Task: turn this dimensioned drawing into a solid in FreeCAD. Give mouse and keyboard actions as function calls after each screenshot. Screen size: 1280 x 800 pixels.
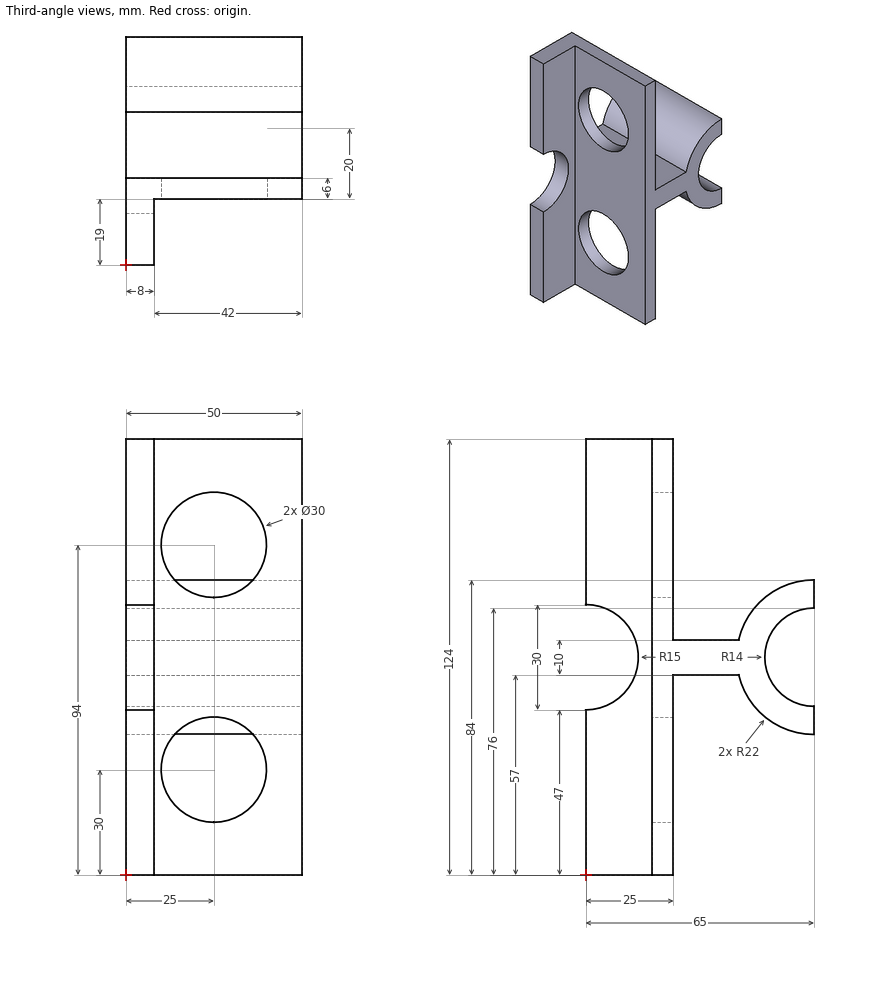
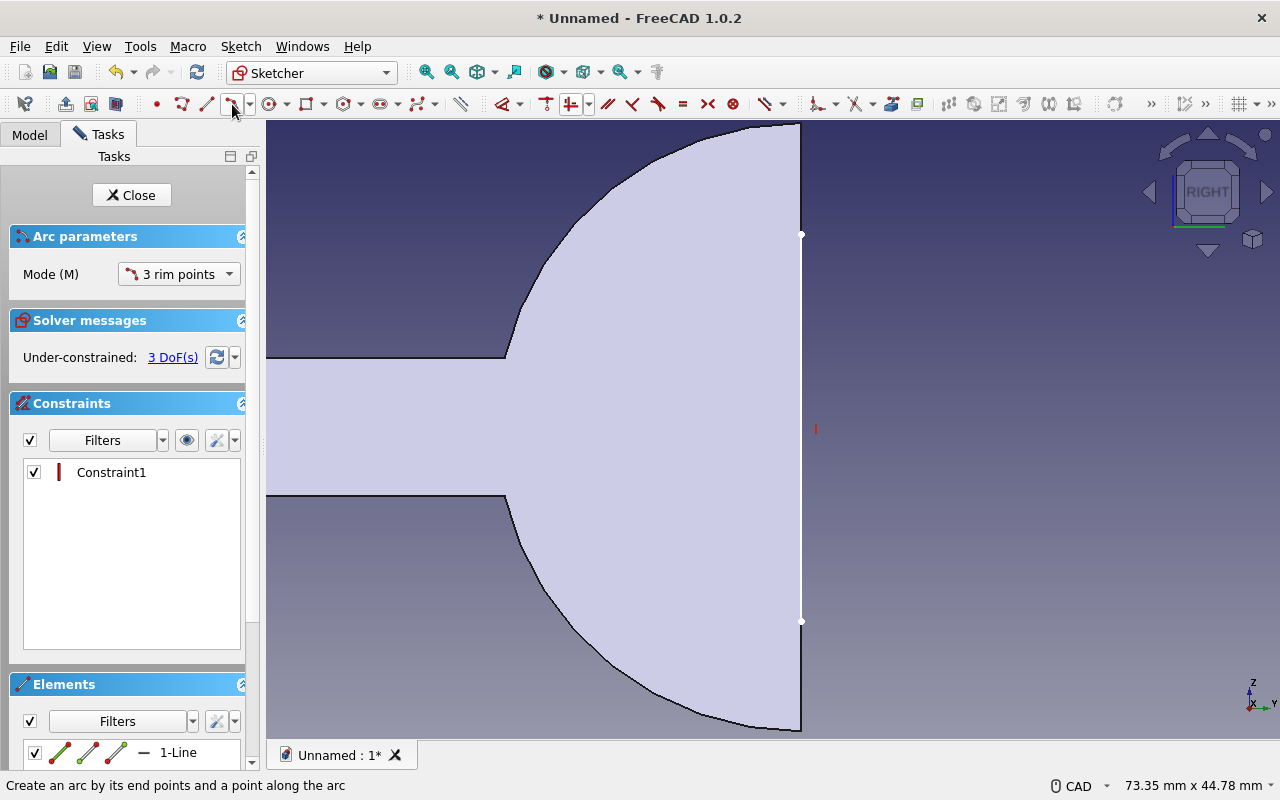
click(801, 622)
click(801, 235)
click(607, 427)
key(Escape)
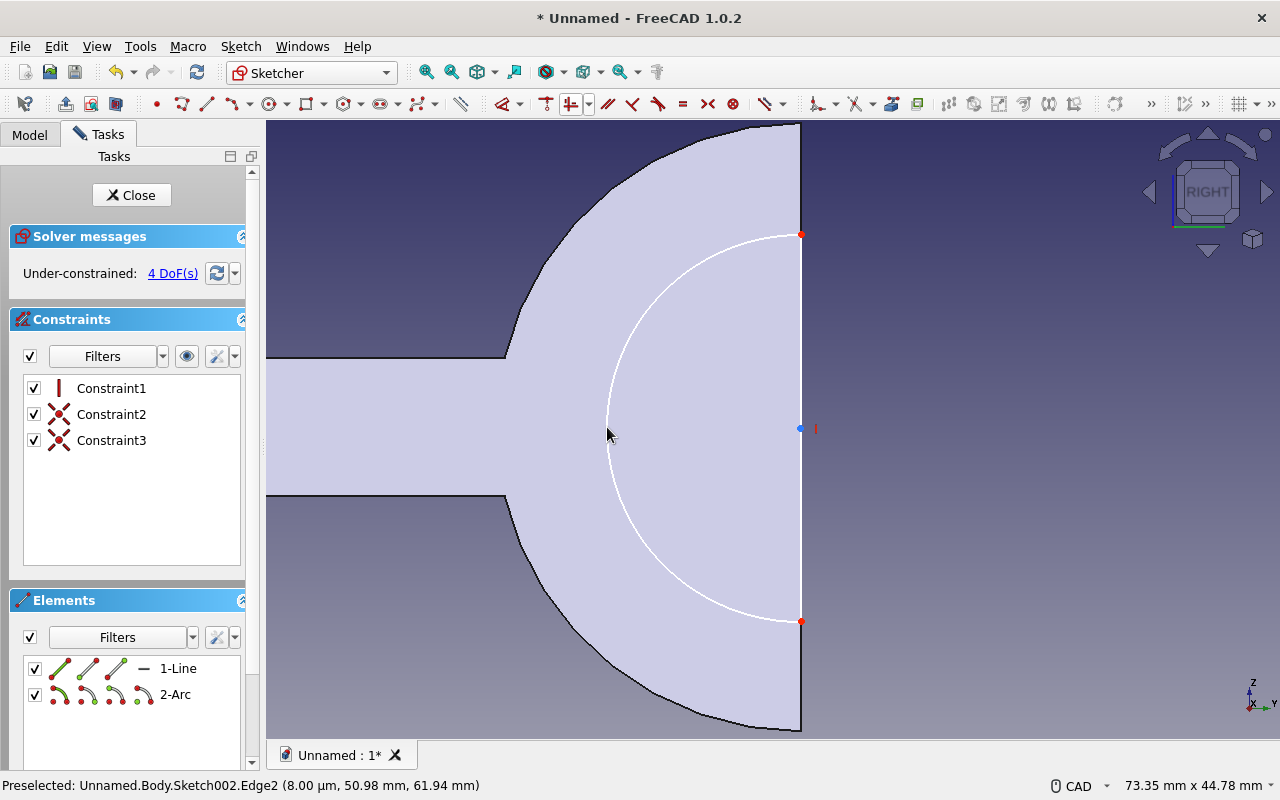
click(502, 104)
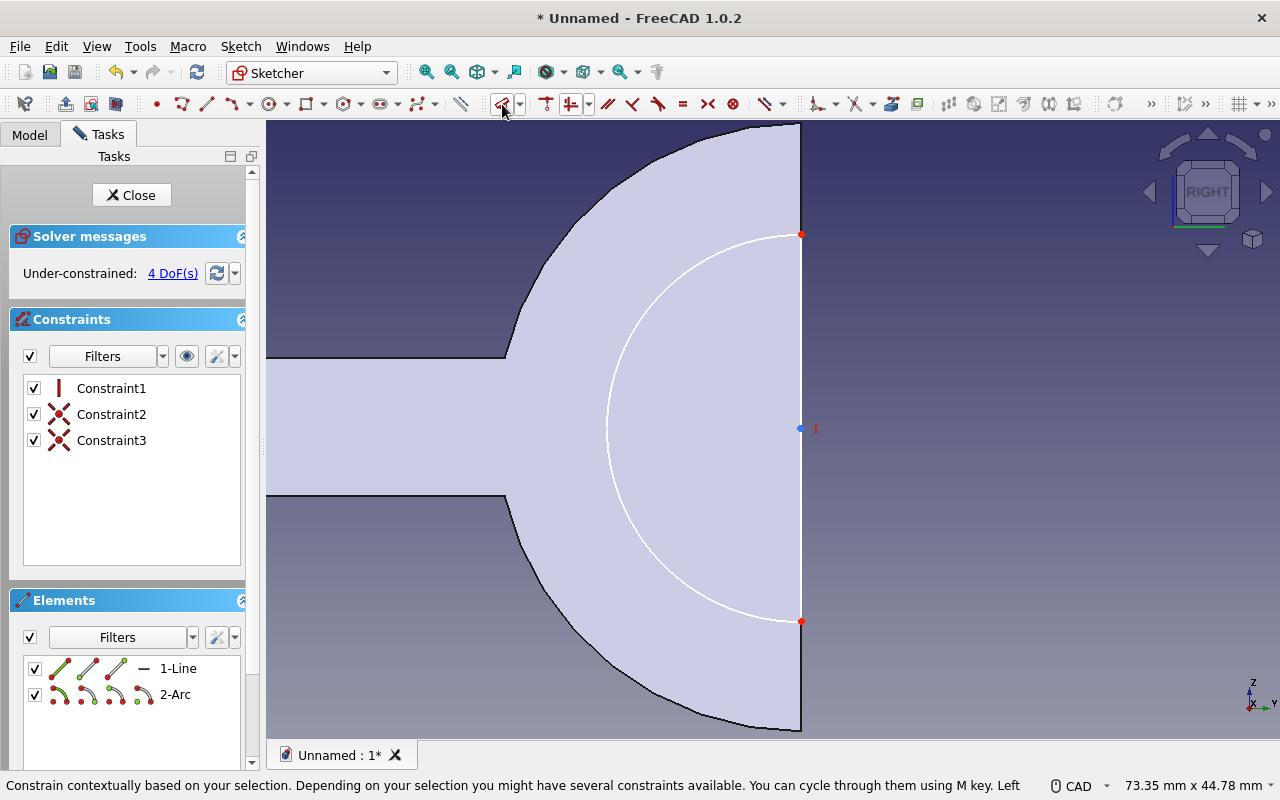
click(644, 315)
click(618, 296)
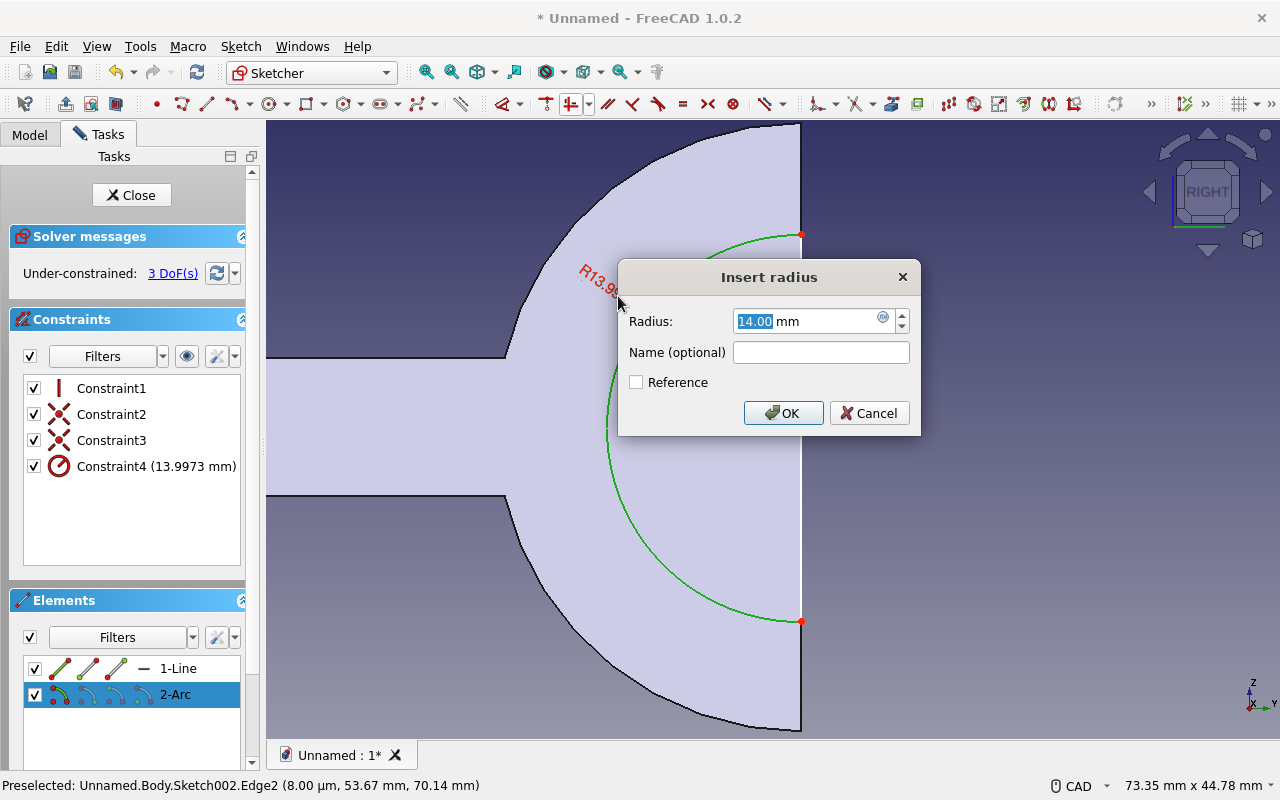
text(14)
key(Return)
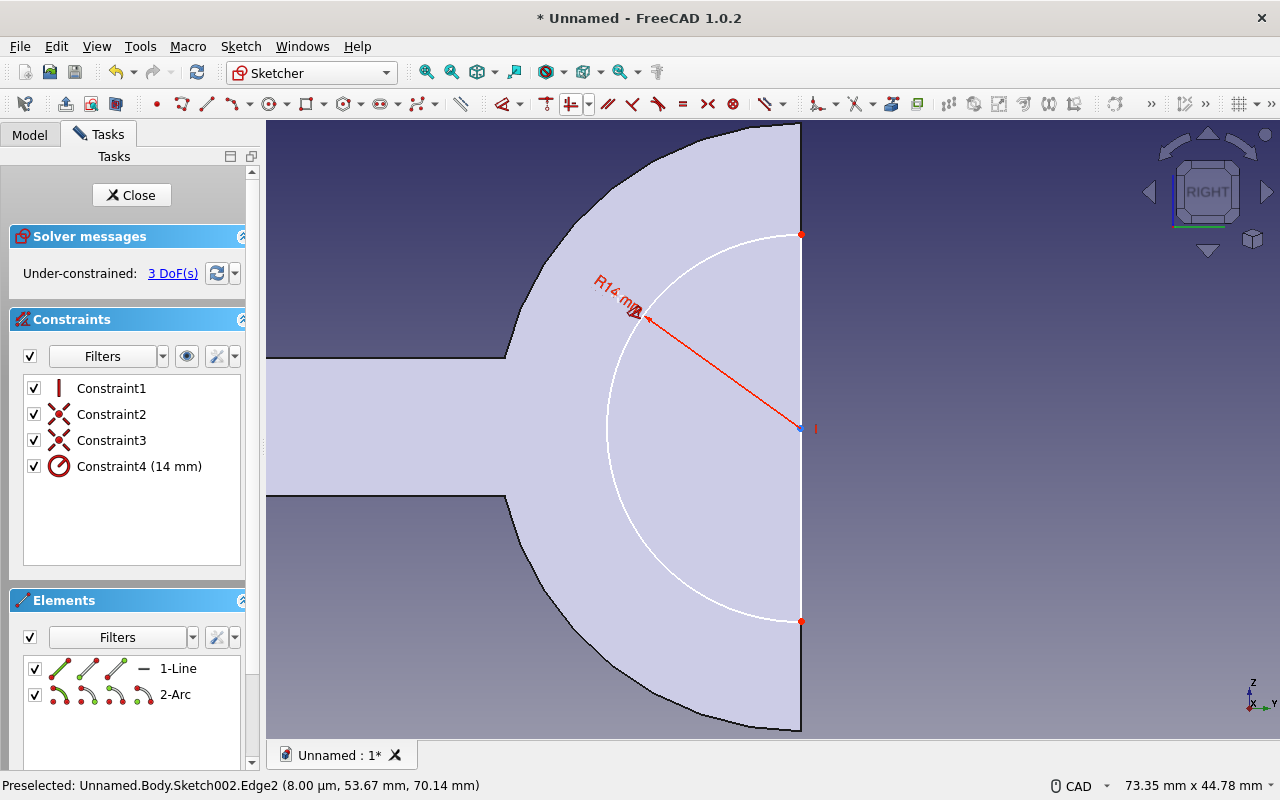
click(801, 235)
click(548, 201)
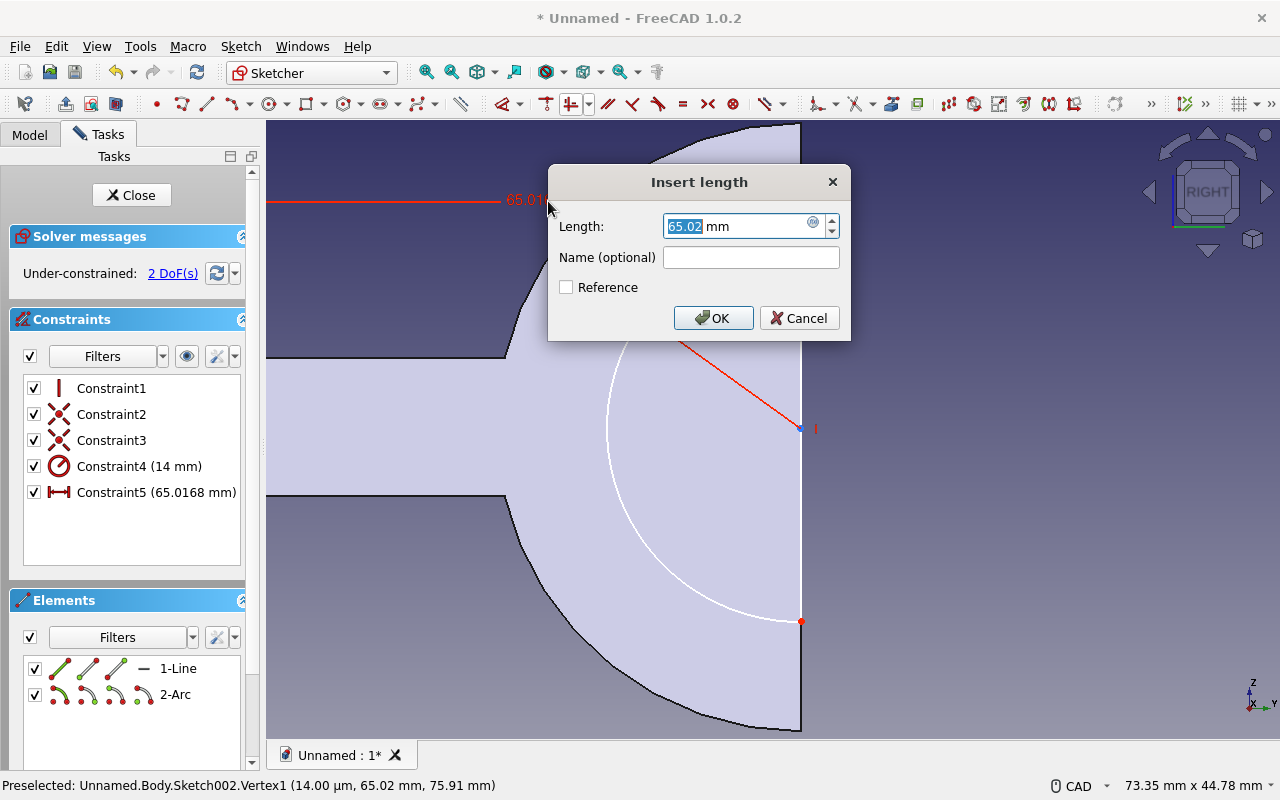
text(65)
key(Return)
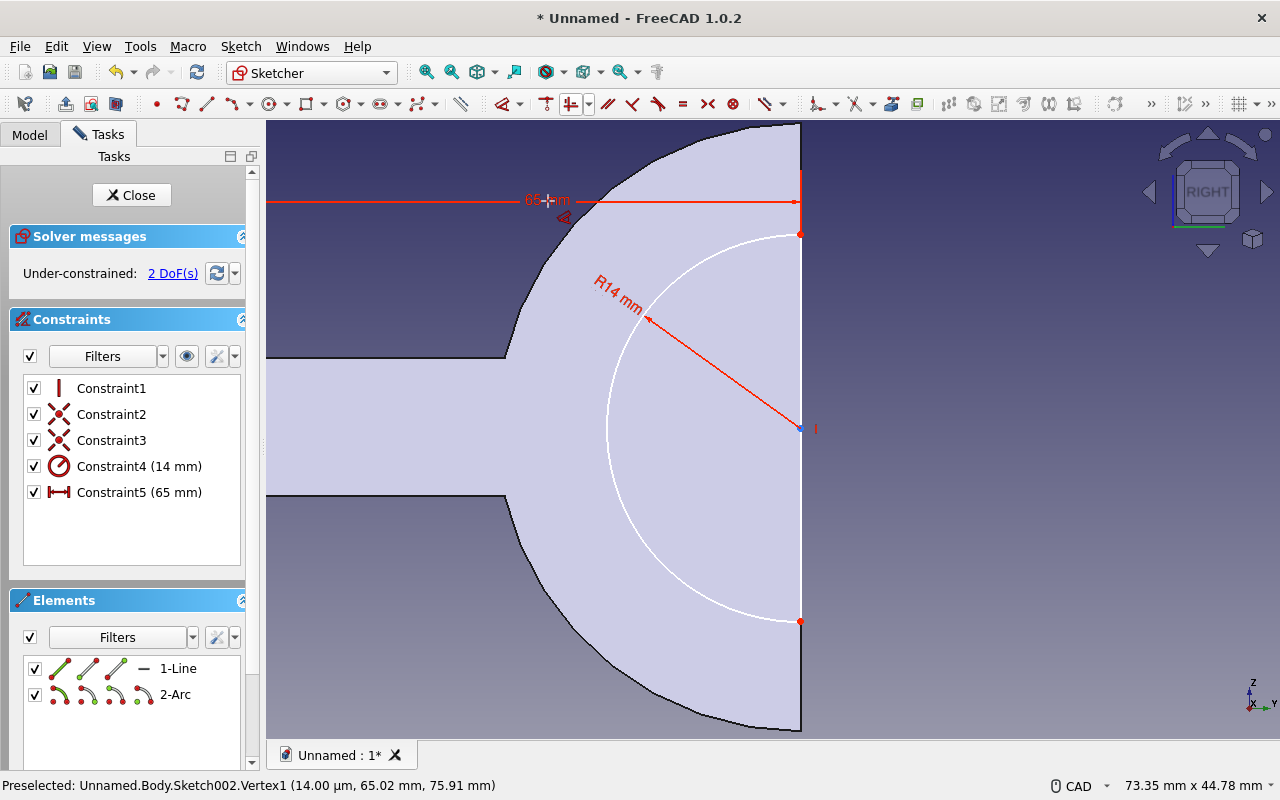
click(801, 235)
click(835, 473)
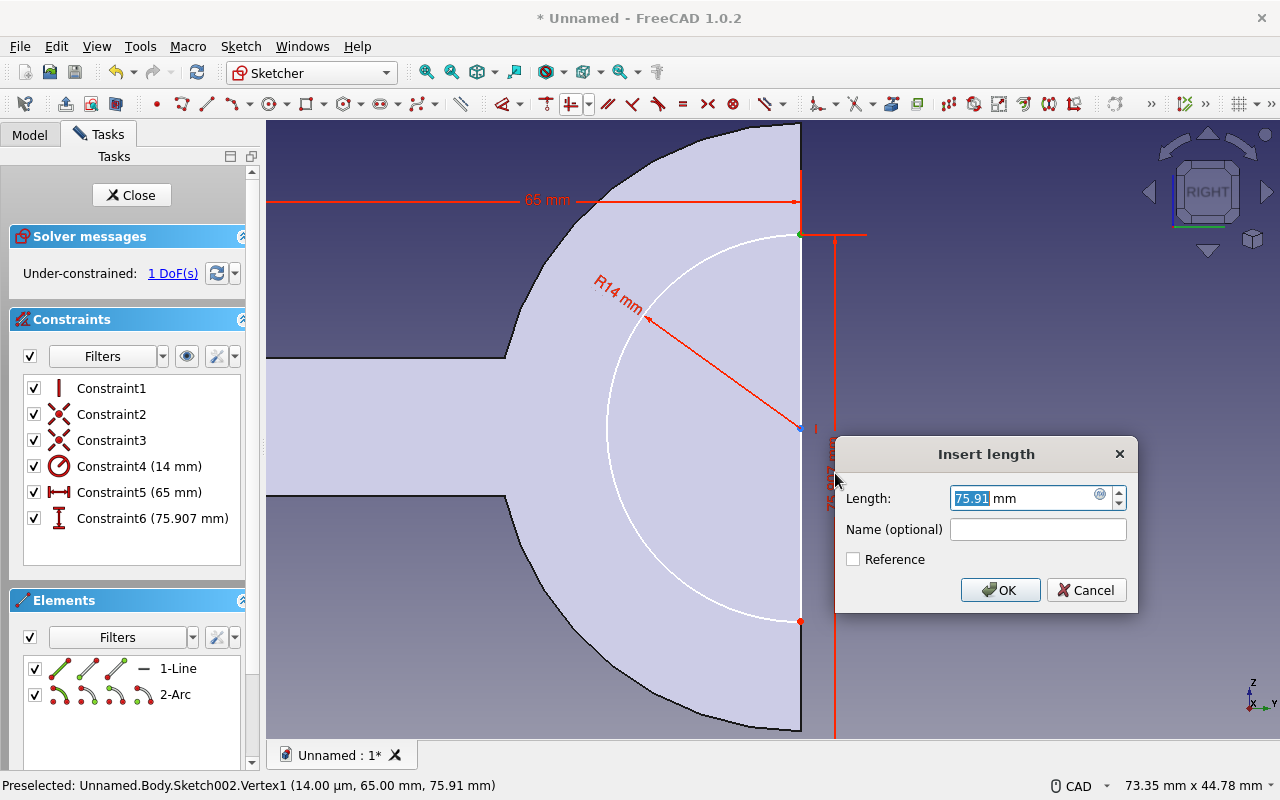
text(76)
key(Return)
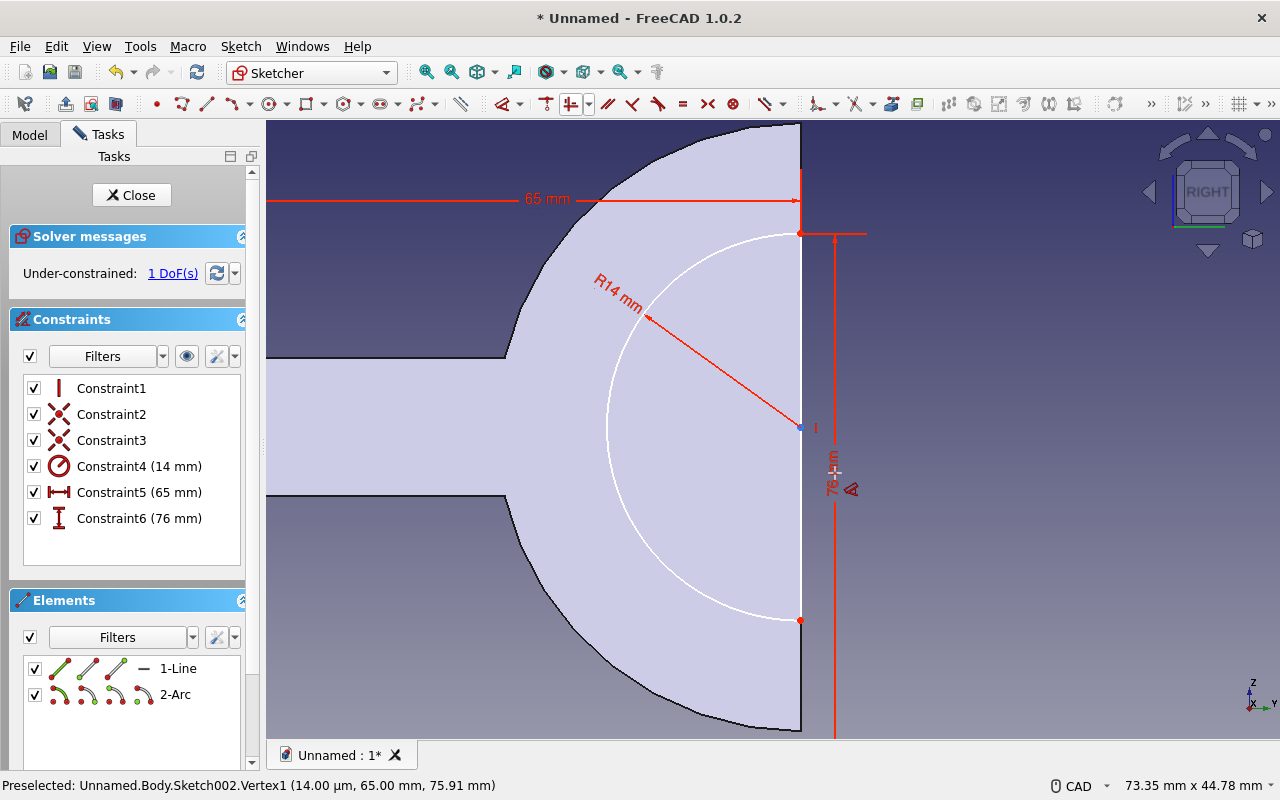
click(801, 427)
click(547, 393)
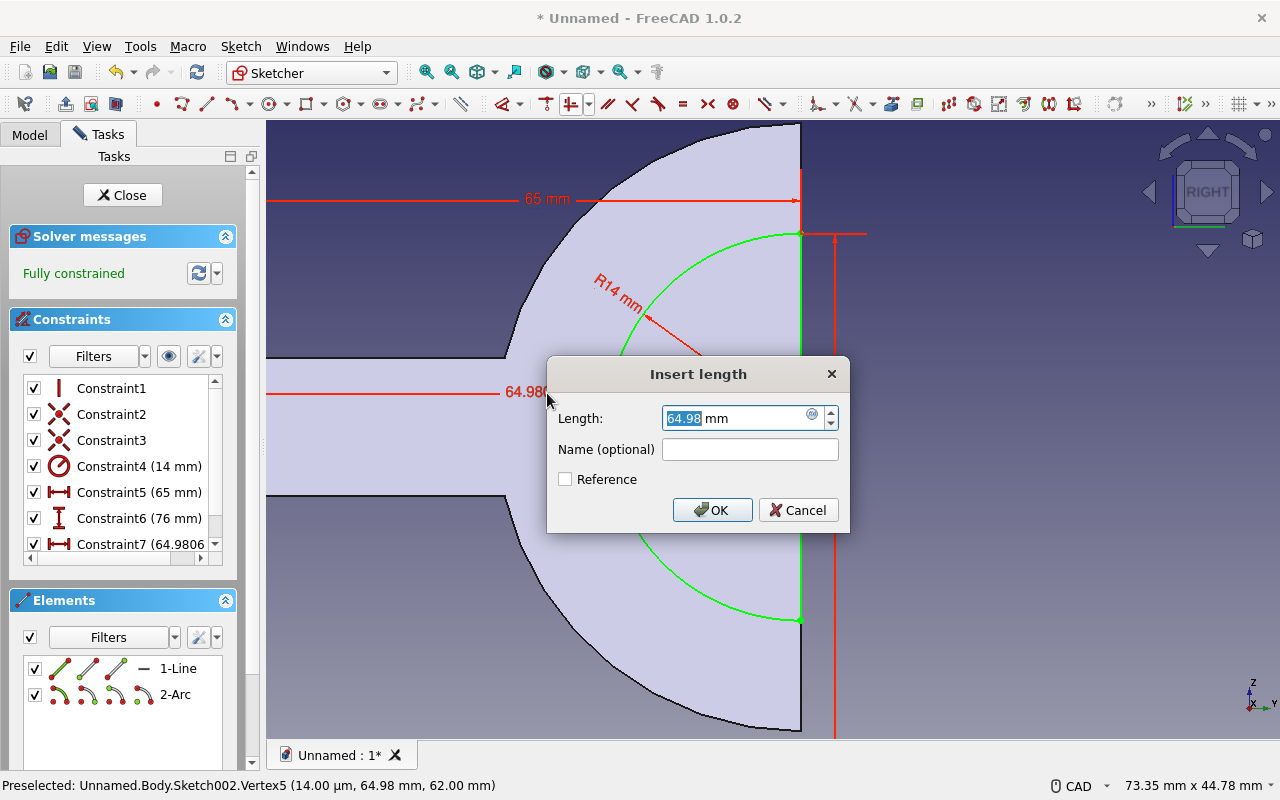
text(65)
key(Return)
key(Escape)